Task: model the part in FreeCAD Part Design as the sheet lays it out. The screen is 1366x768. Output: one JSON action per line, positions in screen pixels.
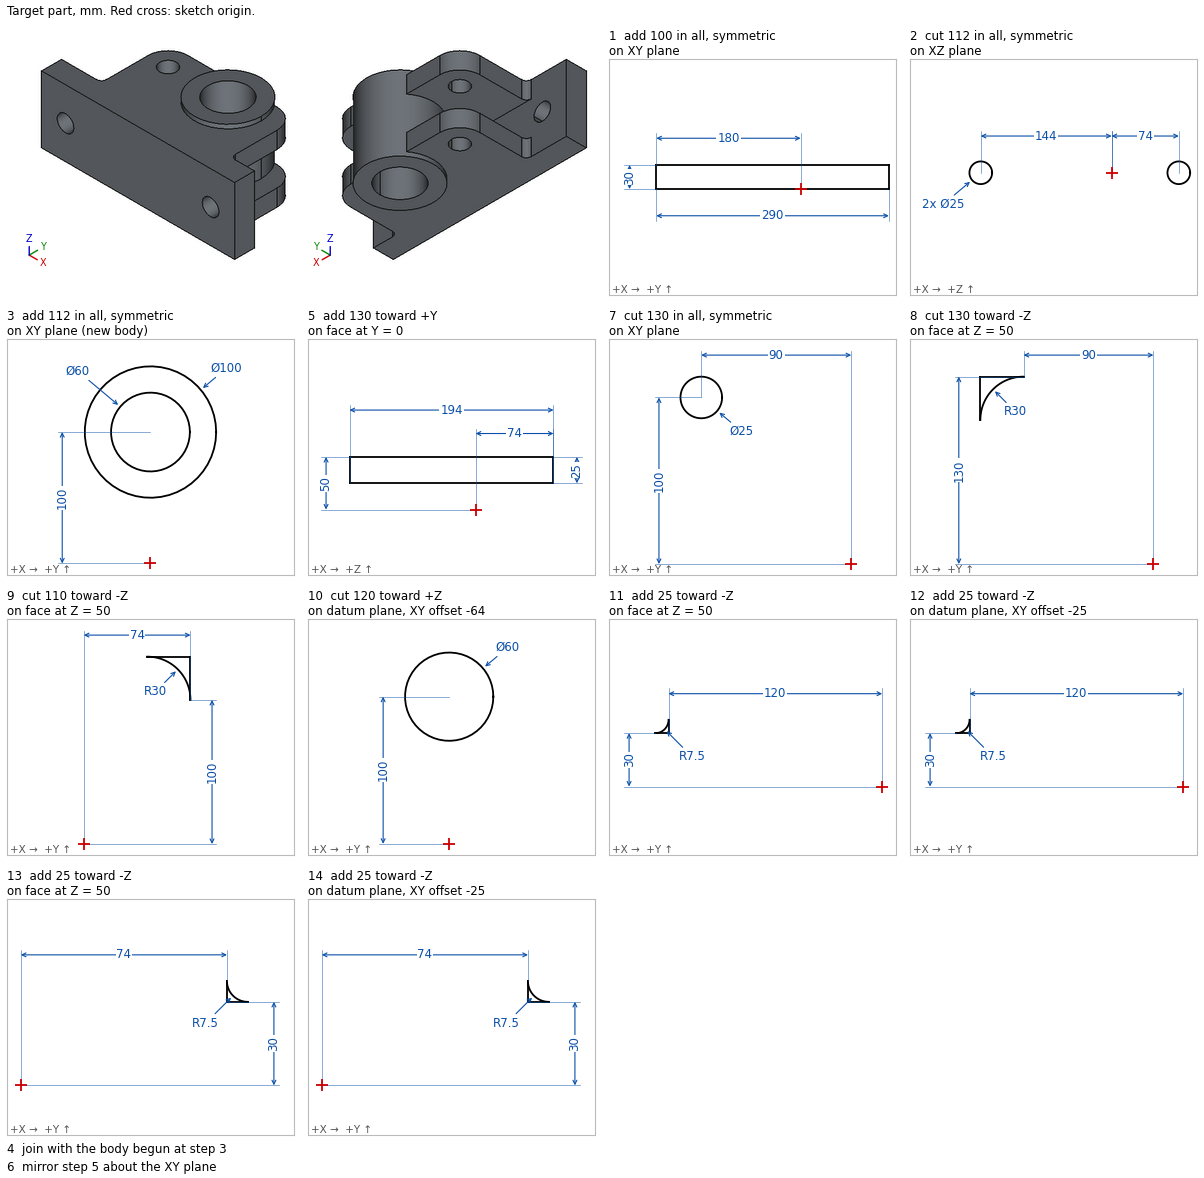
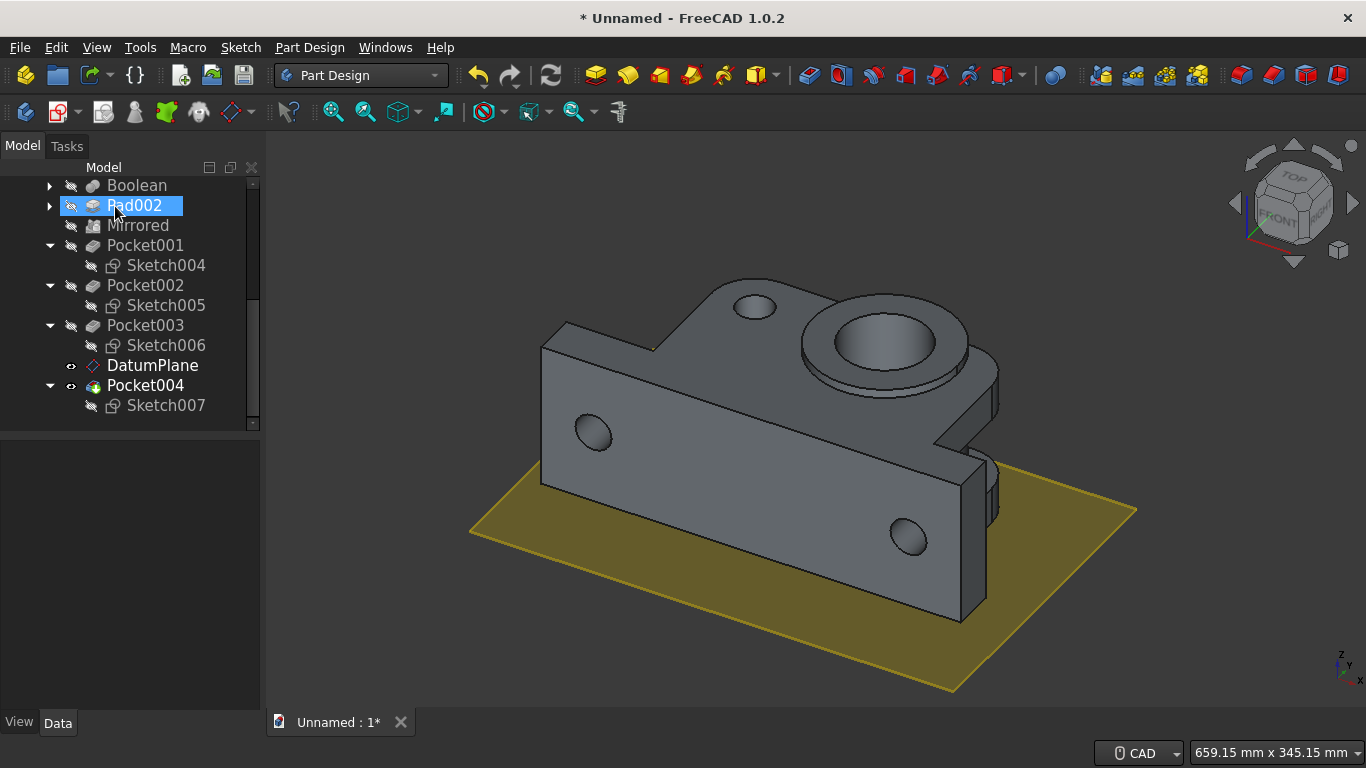
{"action": "left_click", "coordinate": [116, 366]}
{"action": "key", "text": "space"}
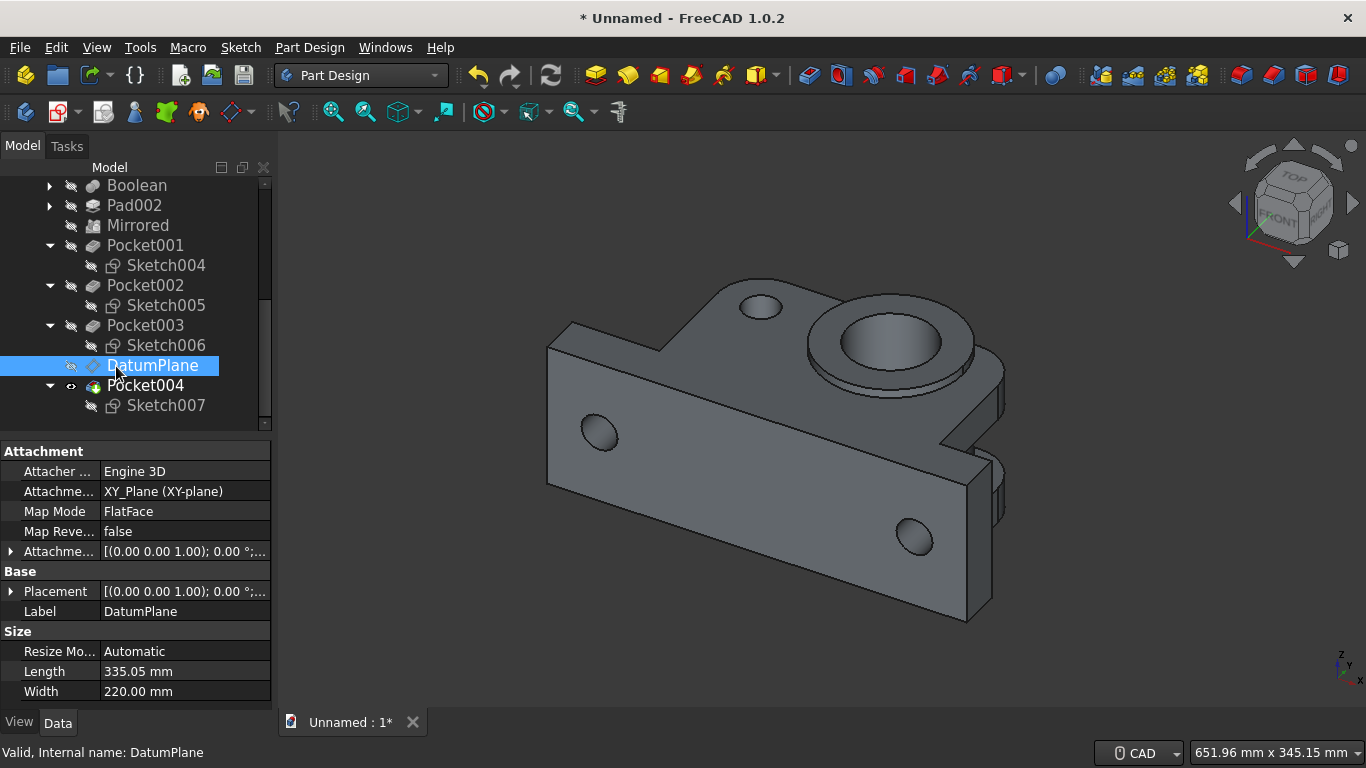
{"action": "left_click", "coordinate": [736, 357]}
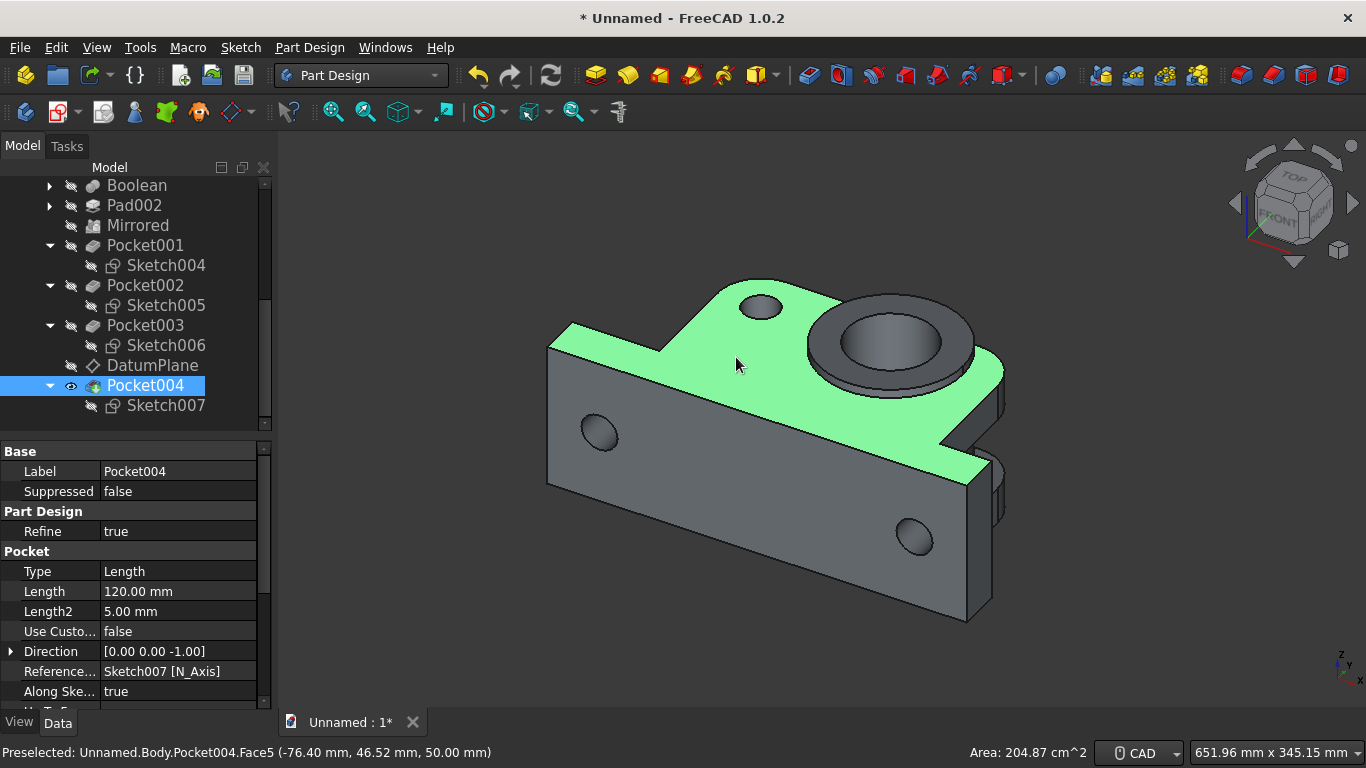
{"action": "left_click", "coordinate": [58, 112]}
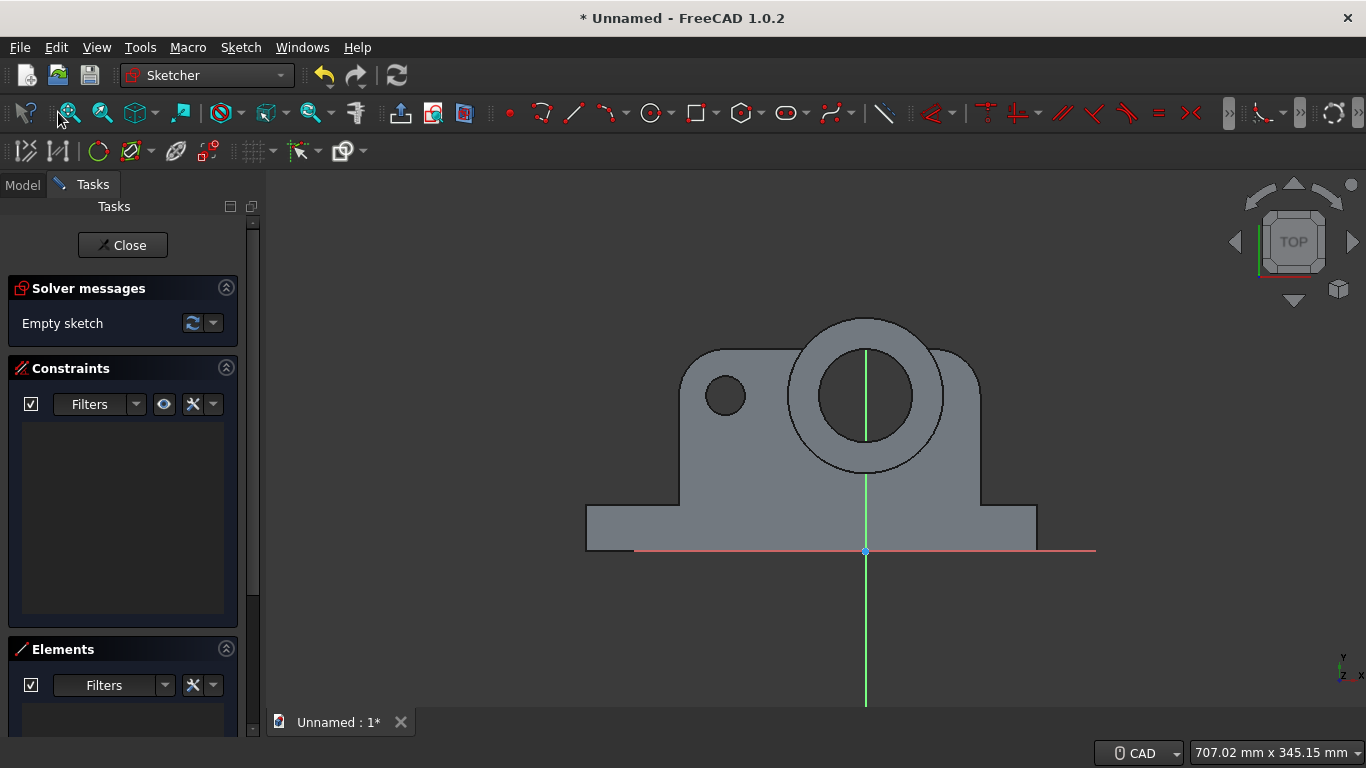
{"action": "scroll", "coordinate": [669, 502], "scroll_direction": "up", "scroll_amount": 15}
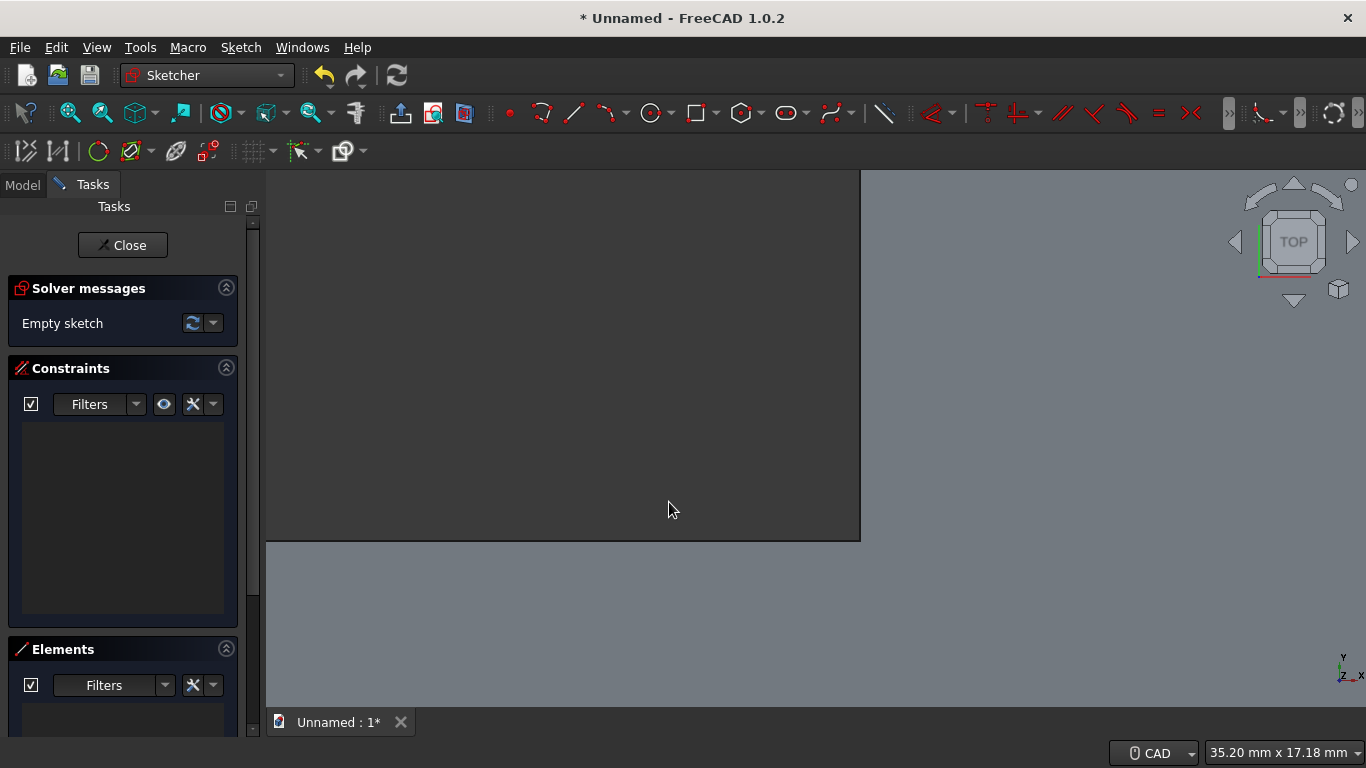
{"action": "scroll", "coordinate": [734, 393], "scroll_direction": "up", "scroll_amount": 2}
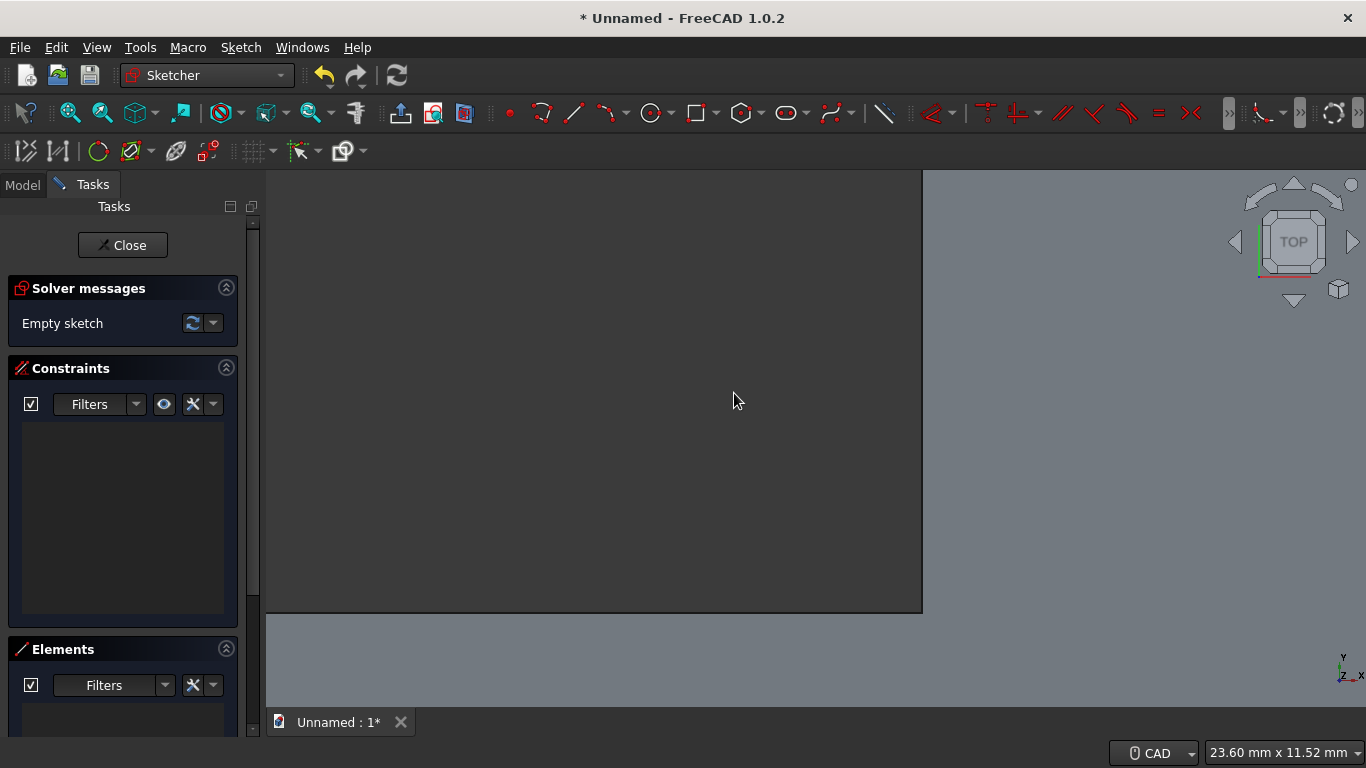
{"action": "left_click", "coordinate": [542, 114]}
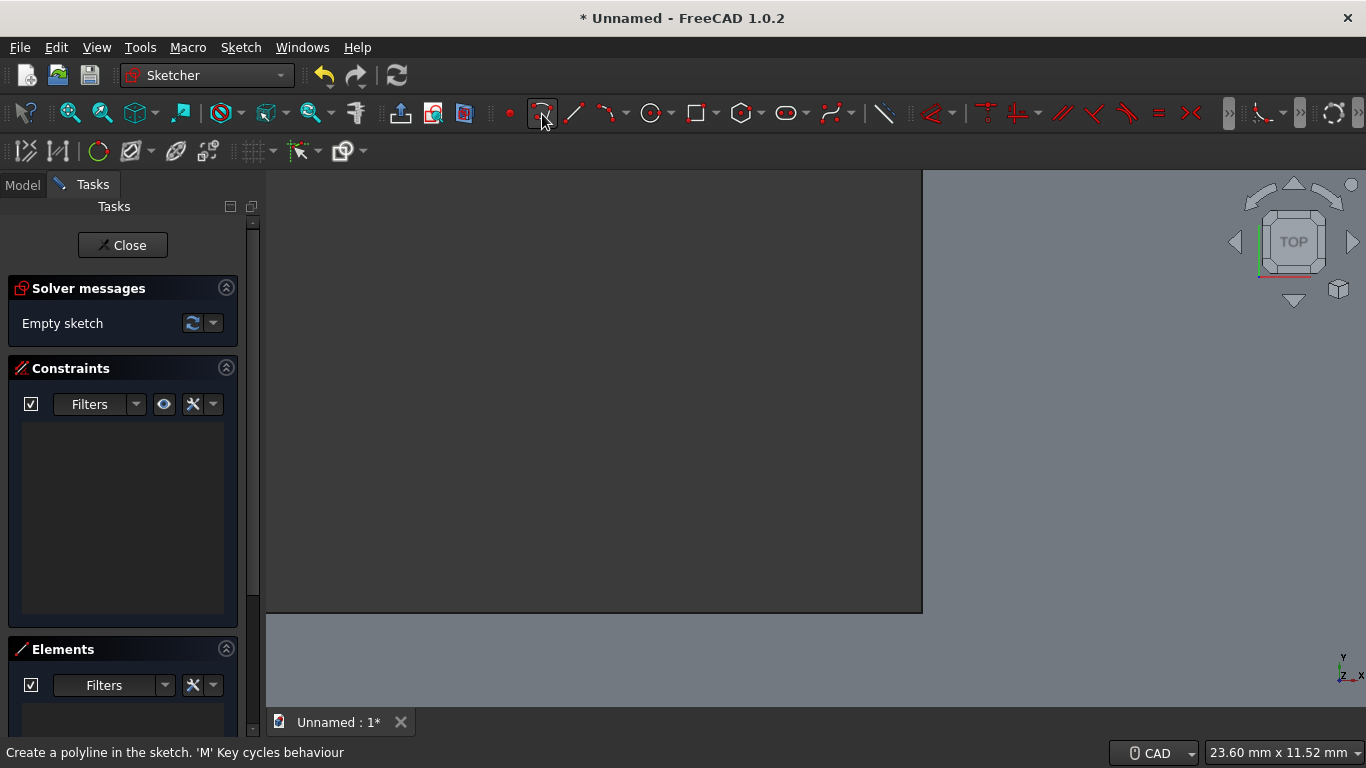
{"action": "left_click", "coordinate": [572, 613]}
{"action": "left_click", "coordinate": [922, 613]}
{"action": "left_click", "coordinate": [922, 264]}
{"action": "right_click", "coordinate": [922, 264]}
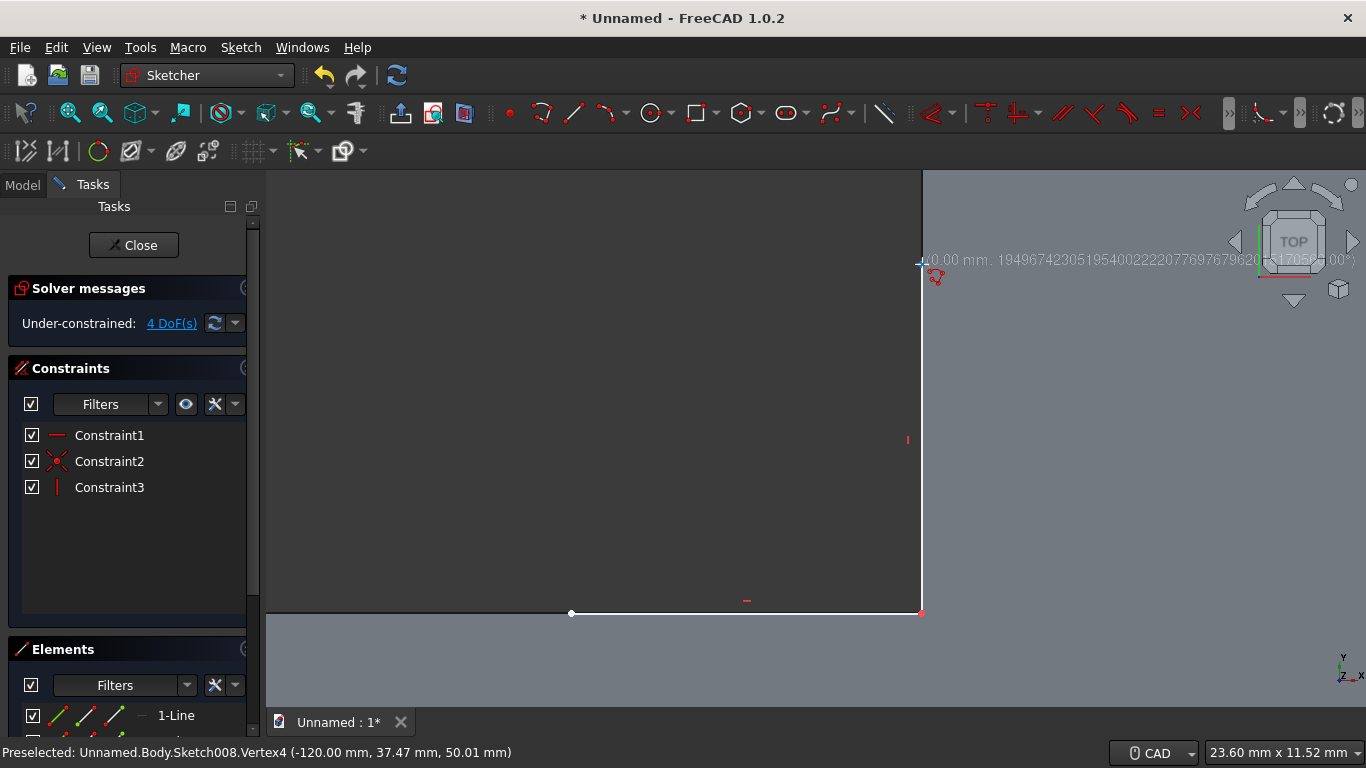
{"action": "left_click", "coordinate": [606, 114]}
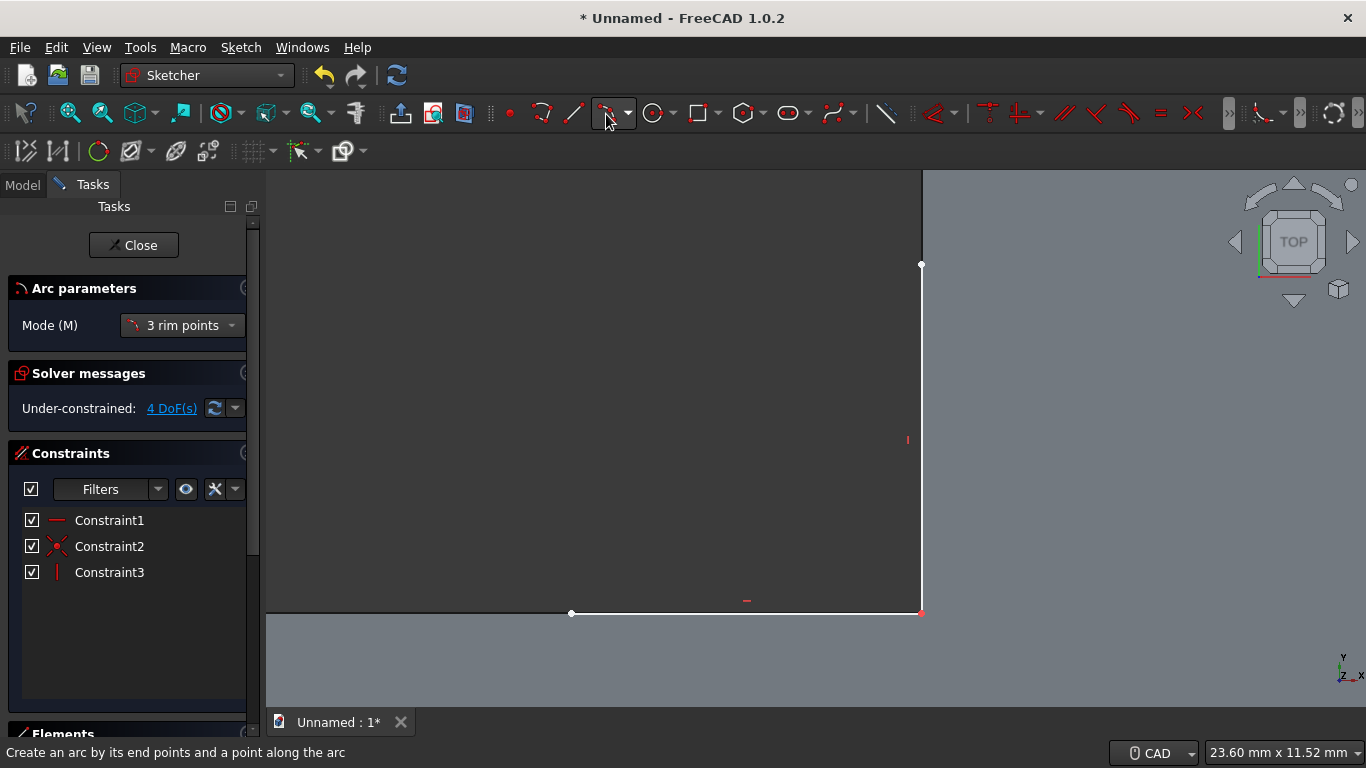
{"action": "left_click", "coordinate": [922, 265]}
{"action": "left_click", "coordinate": [572, 614]}
{"action": "left_click", "coordinate": [820, 511]}
{"action": "key", "text": "Escape"}